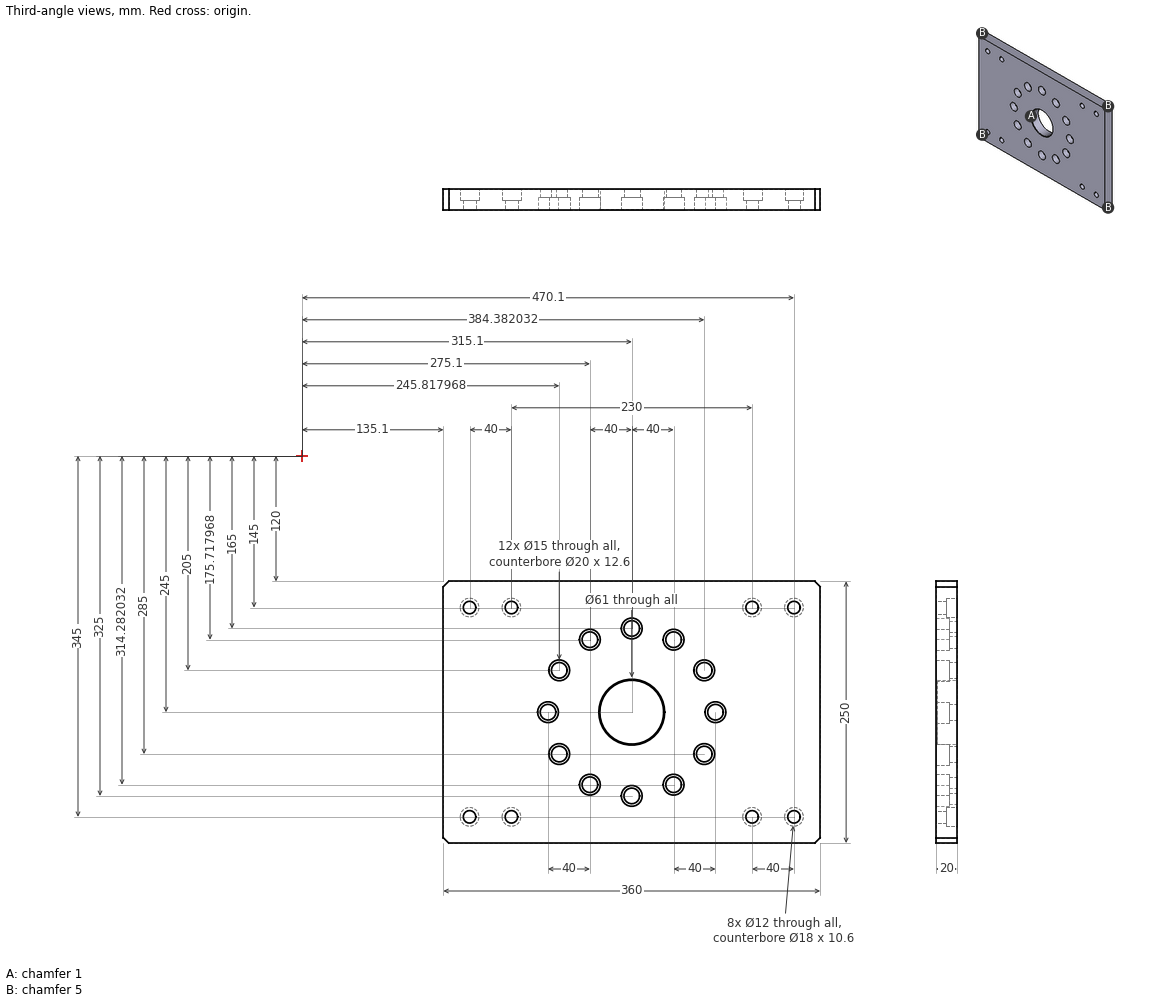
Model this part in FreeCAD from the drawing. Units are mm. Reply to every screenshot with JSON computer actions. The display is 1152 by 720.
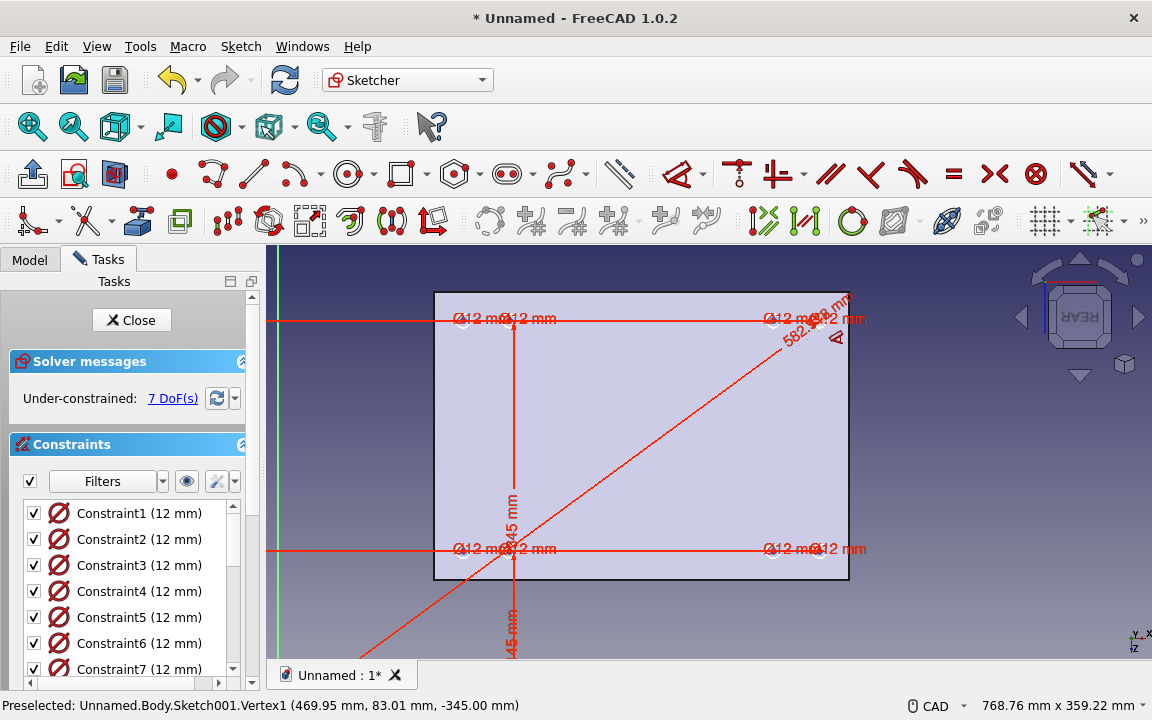
{"action": "left_click", "coordinate": [773, 321]}
{"action": "left_click", "coordinate": [797, 287]}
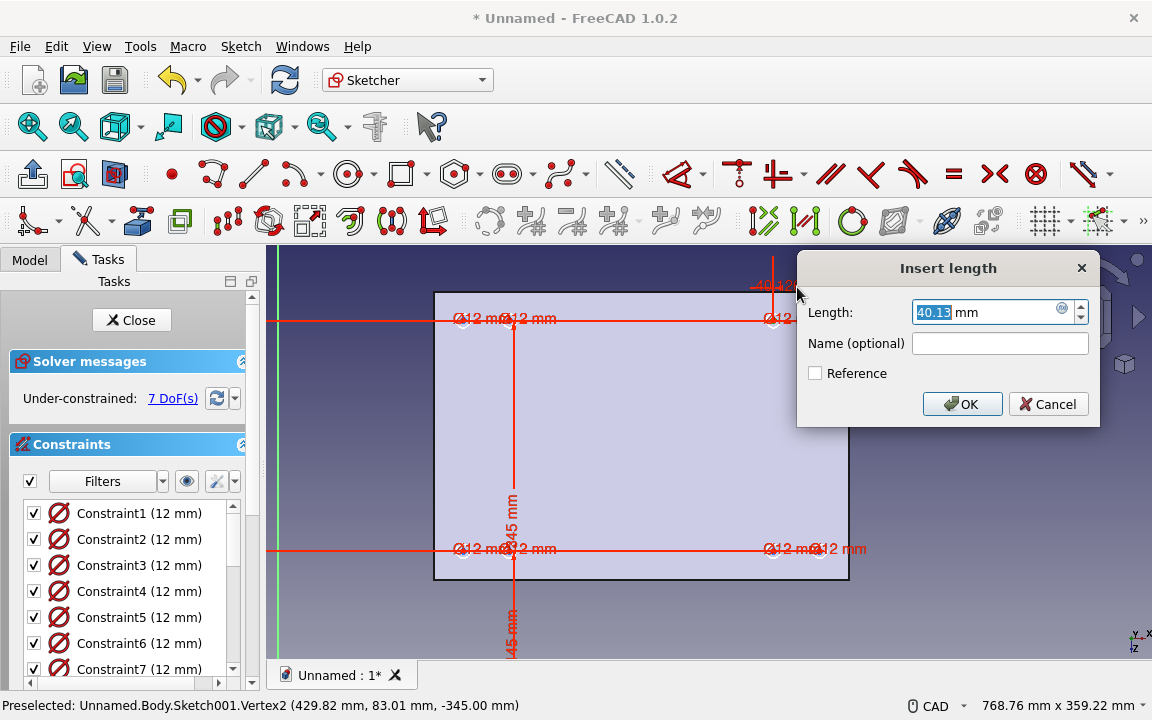
{"action": "type", "text": "40"}
{"action": "key", "text": "Return"}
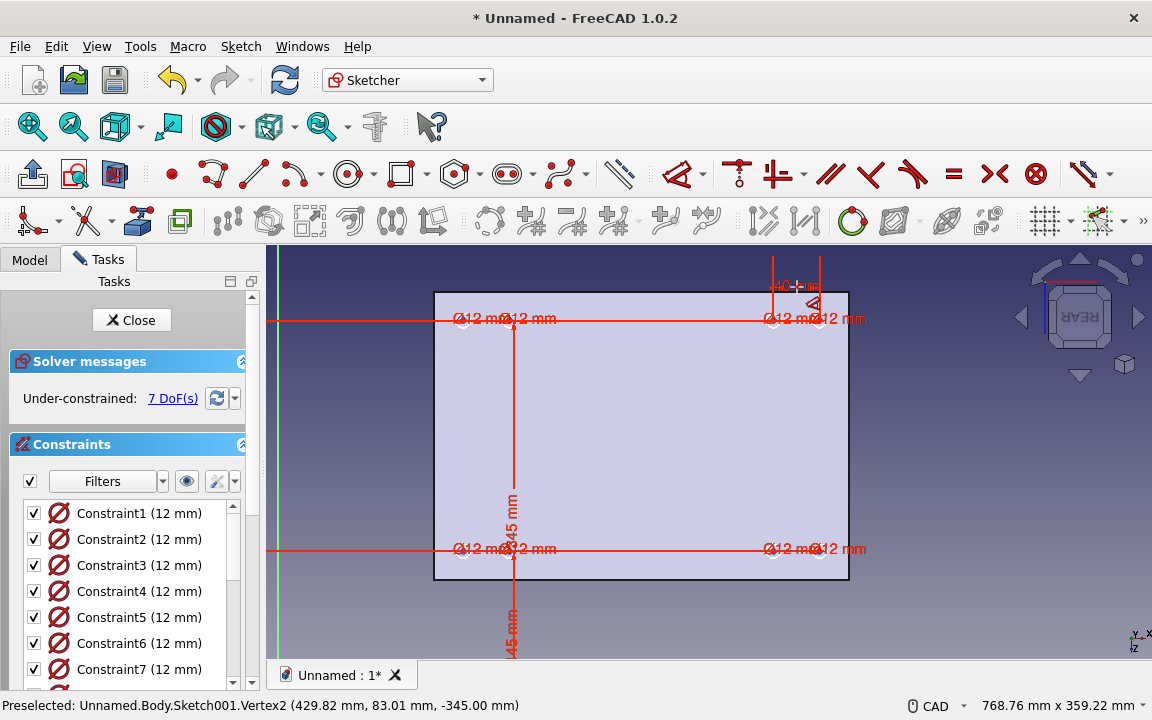
{"action": "left_click", "coordinate": [773, 321]}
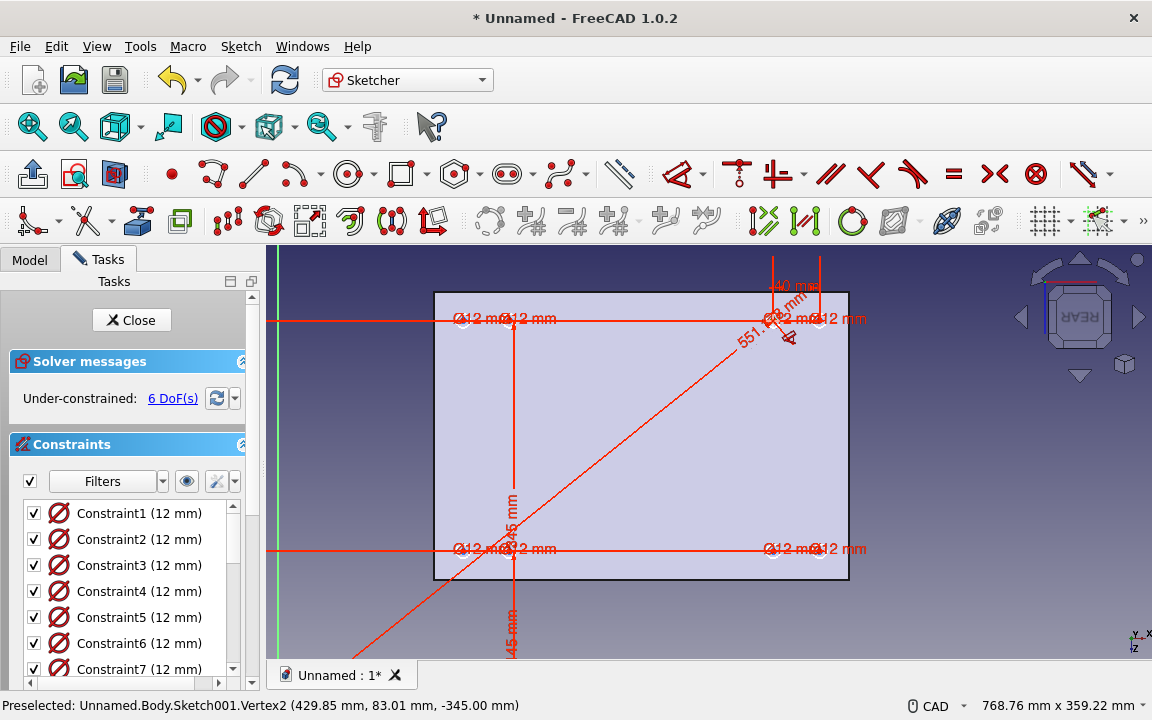
{"action": "left_click", "coordinate": [820, 551]}
{"action": "left_click", "coordinate": [797, 585]}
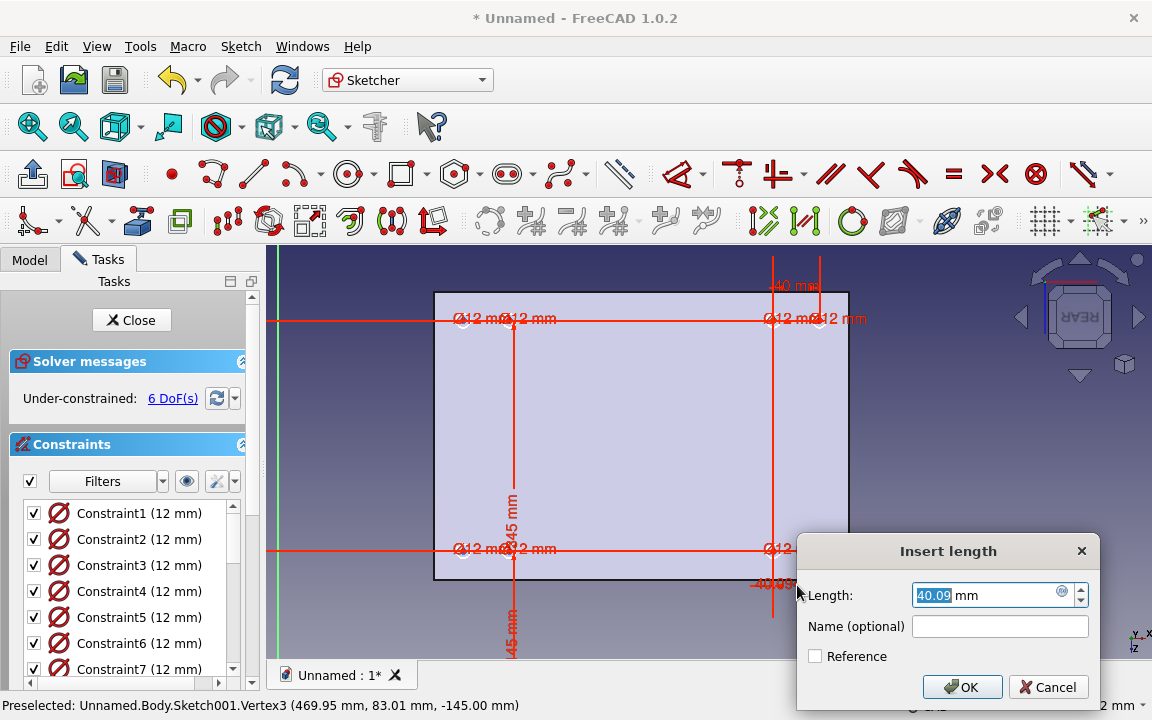
{"action": "type", "text": "40"}
{"action": "key", "text": "Return"}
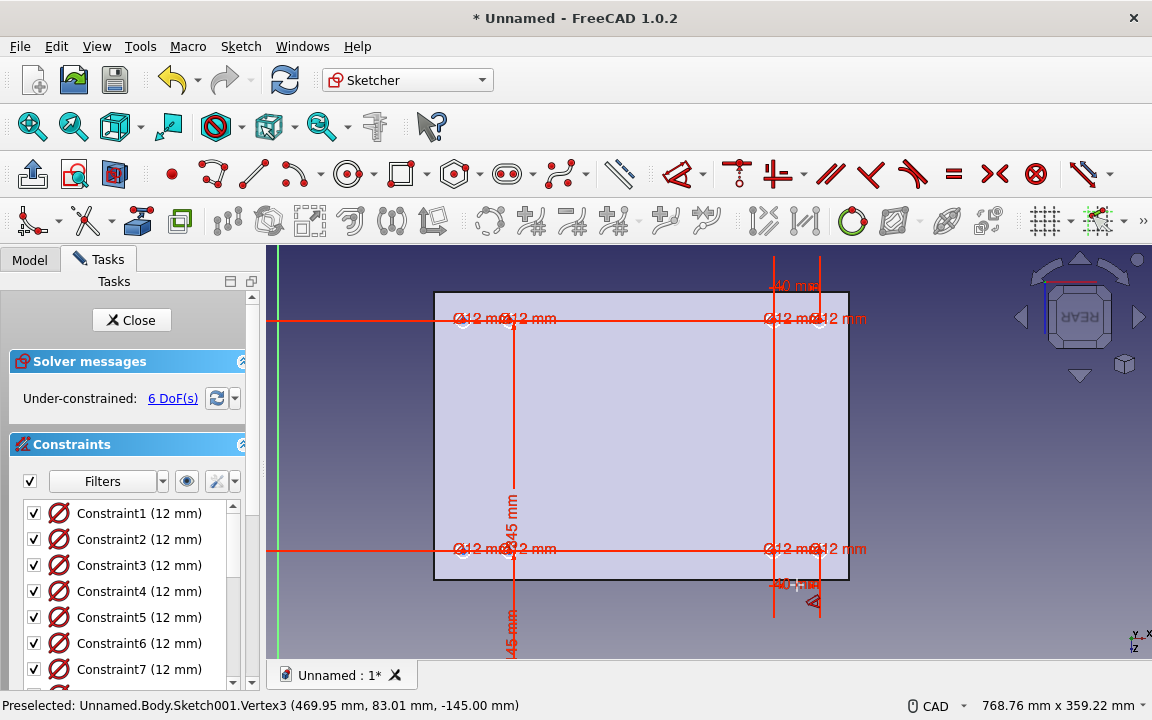
{"action": "left_click", "coordinate": [820, 551]}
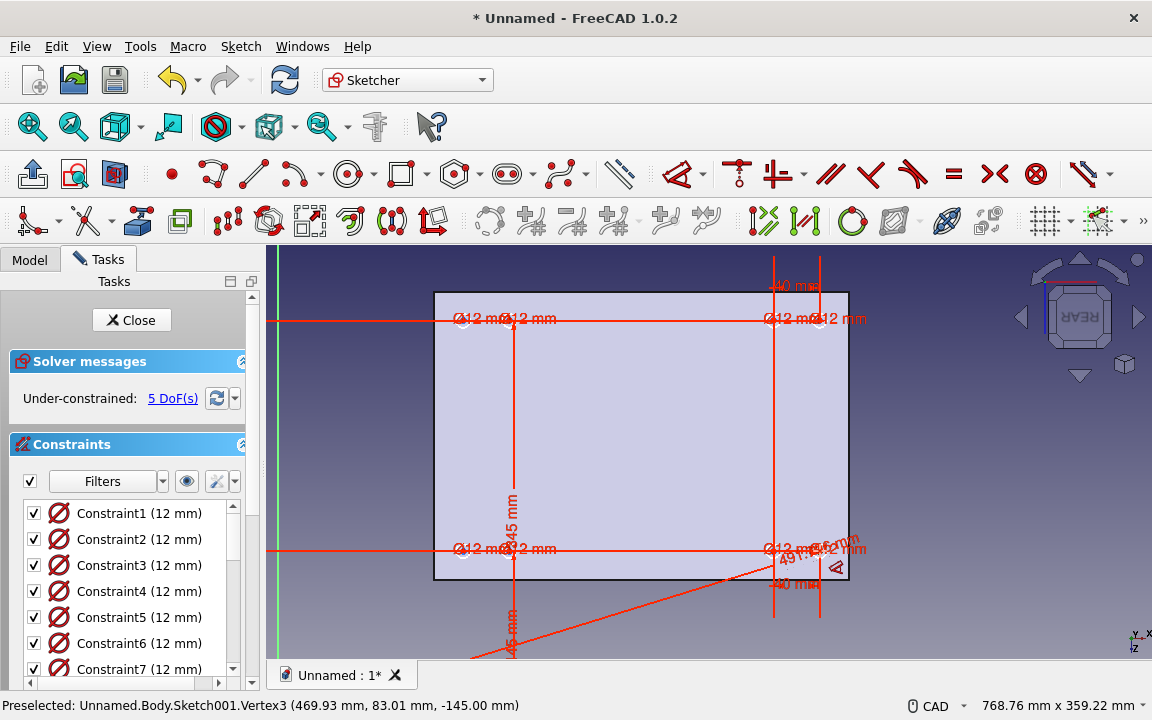
{"action": "left_click", "coordinate": [773, 551]}
{"action": "left_click", "coordinate": [797, 517]}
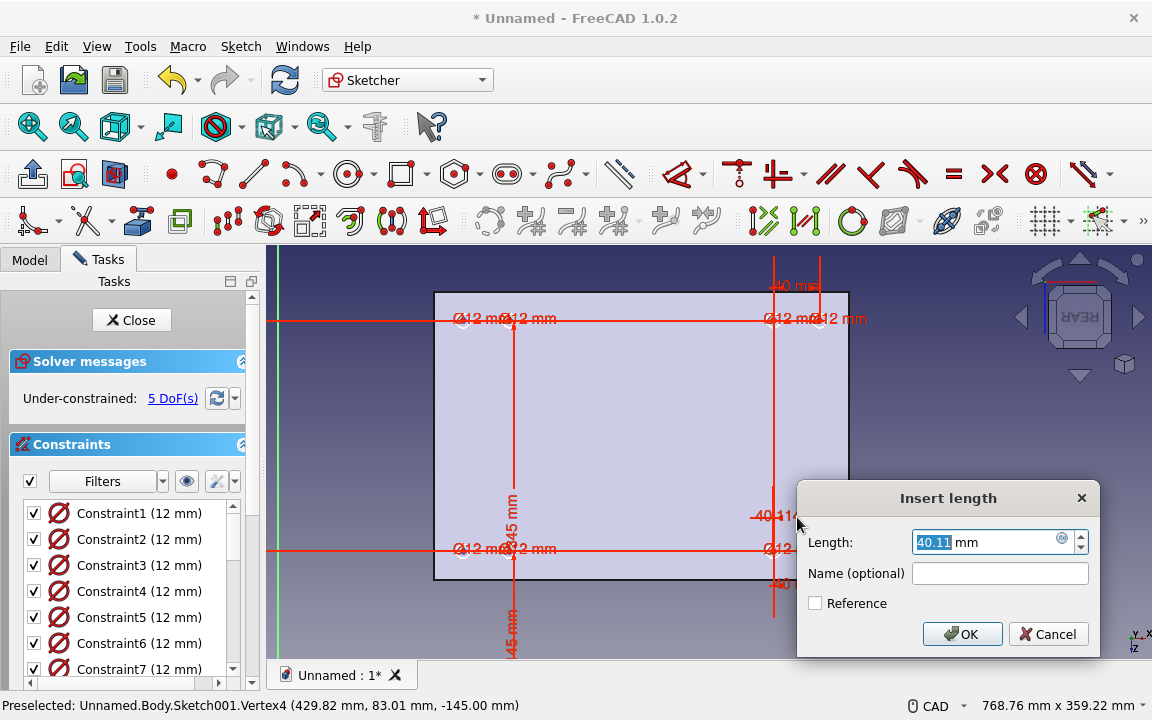
{"action": "type", "text": "40"}
{"action": "key", "text": "Return"}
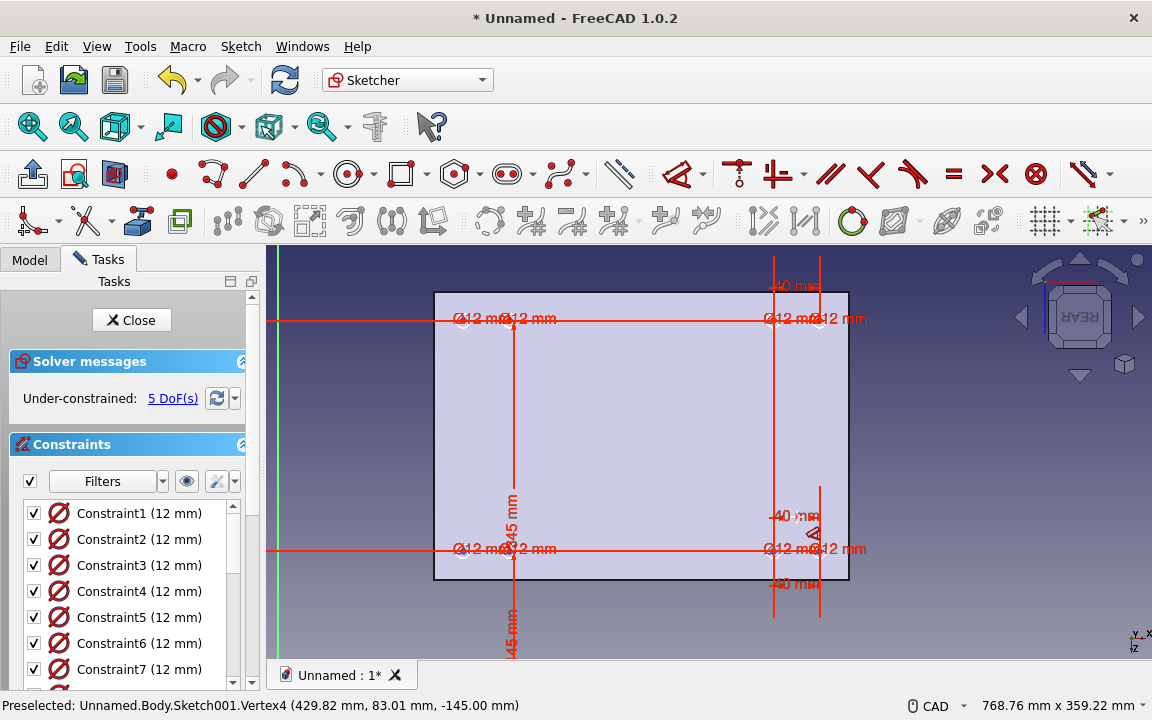
{"action": "left_click", "coordinate": [509, 551]}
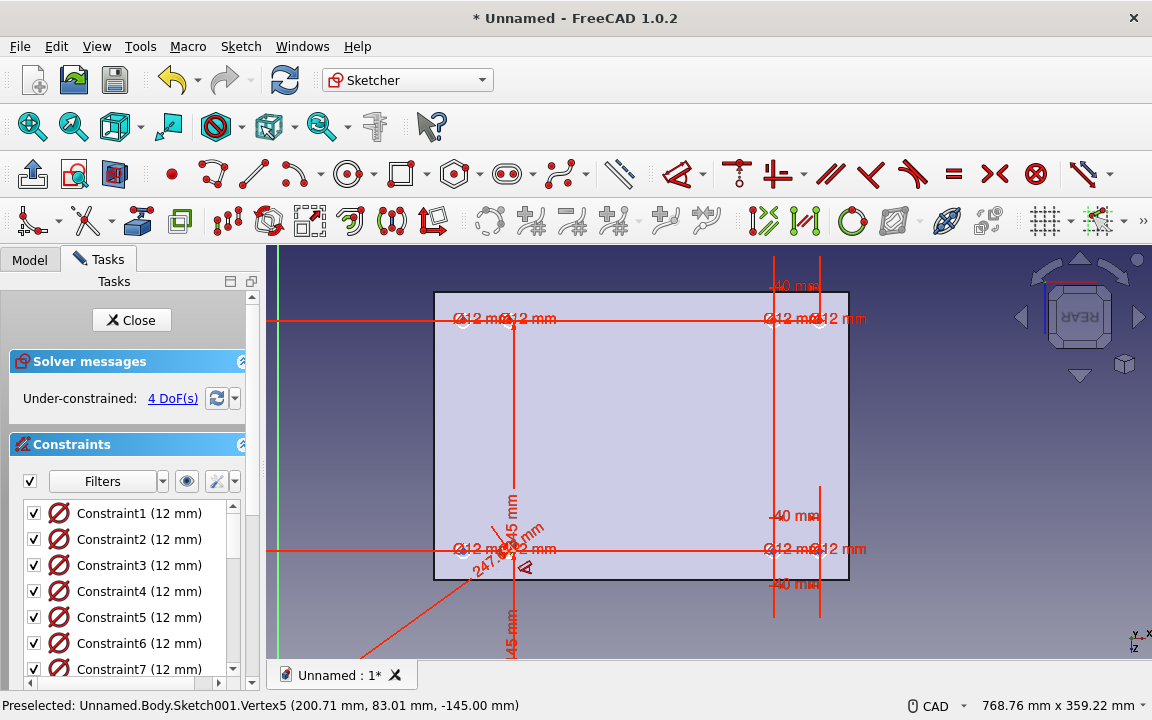
{"action": "left_click", "coordinate": [463, 551]}
{"action": "left_click", "coordinate": [486, 585]}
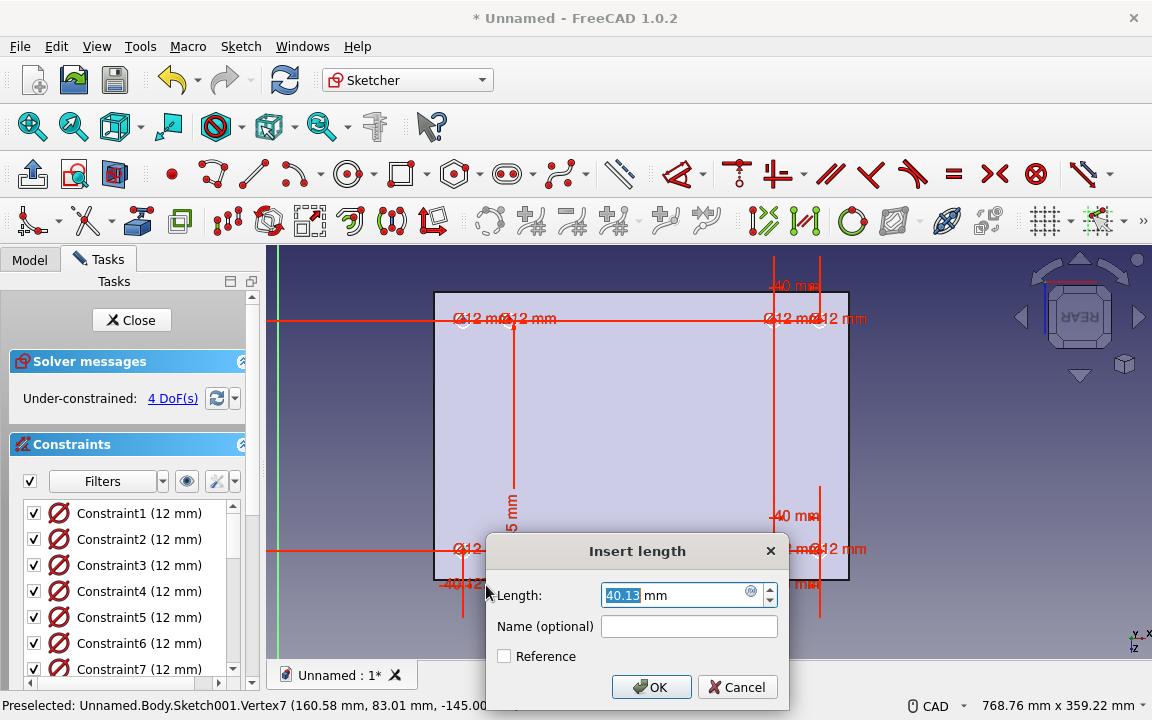
{"action": "type", "text": "40"}
{"action": "key", "text": "Return"}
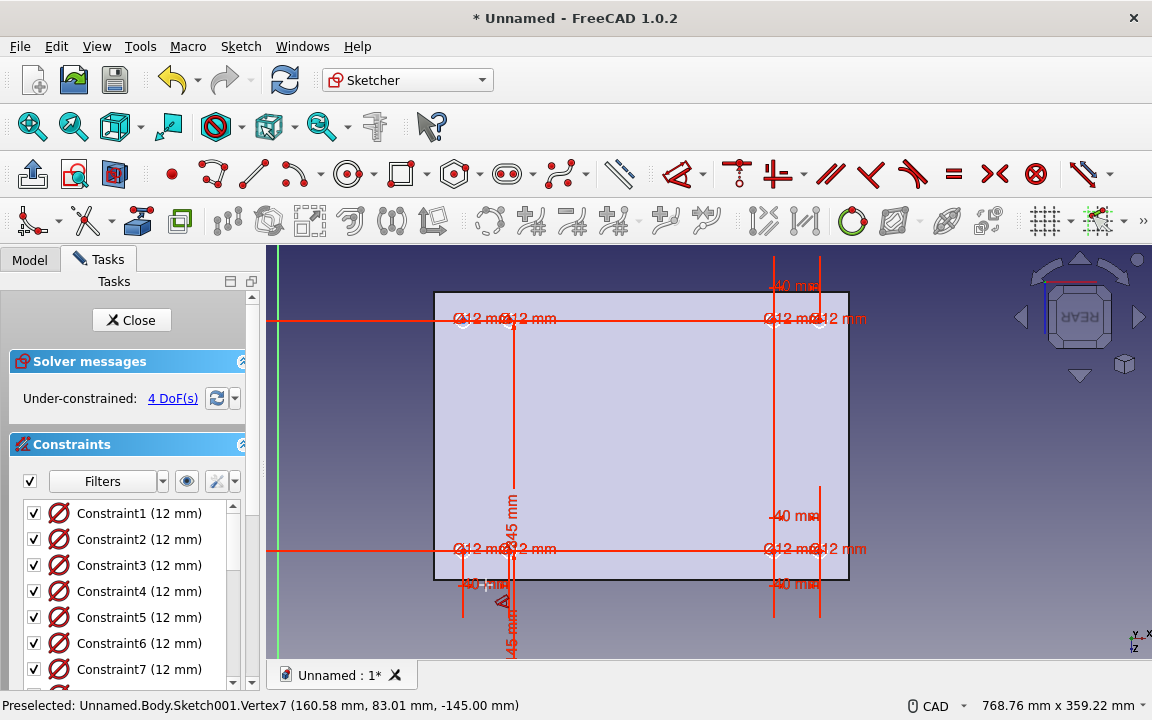
{"action": "left_click", "coordinate": [509, 321]}